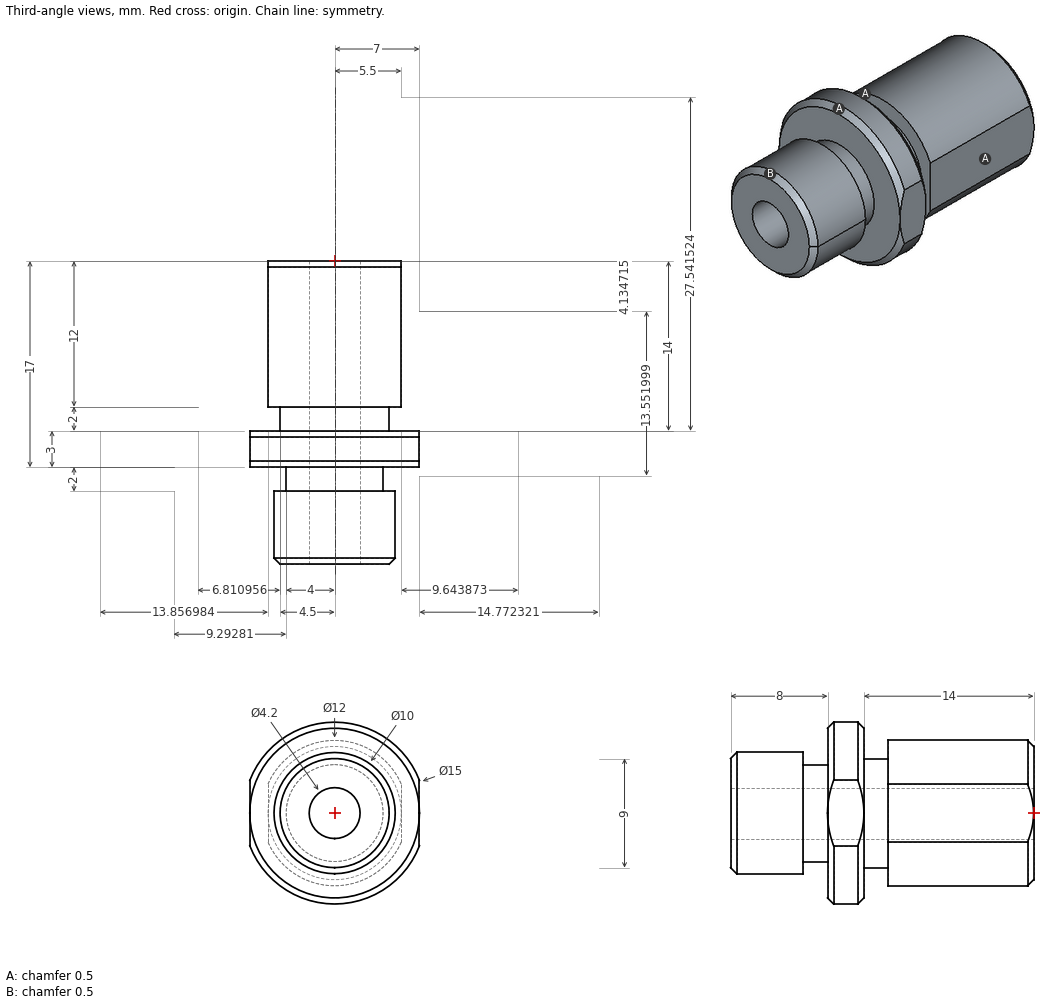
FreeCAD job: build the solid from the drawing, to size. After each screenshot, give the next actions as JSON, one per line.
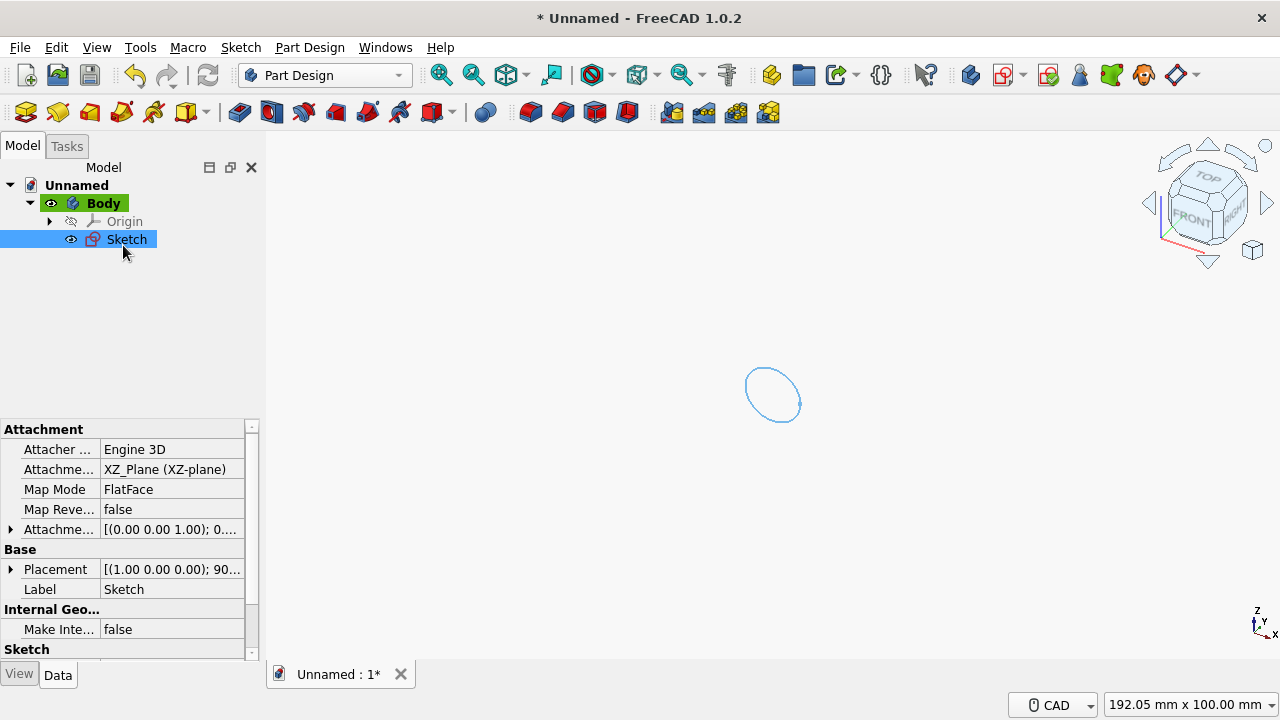
{"action": "left_click", "coordinate": [26, 112]}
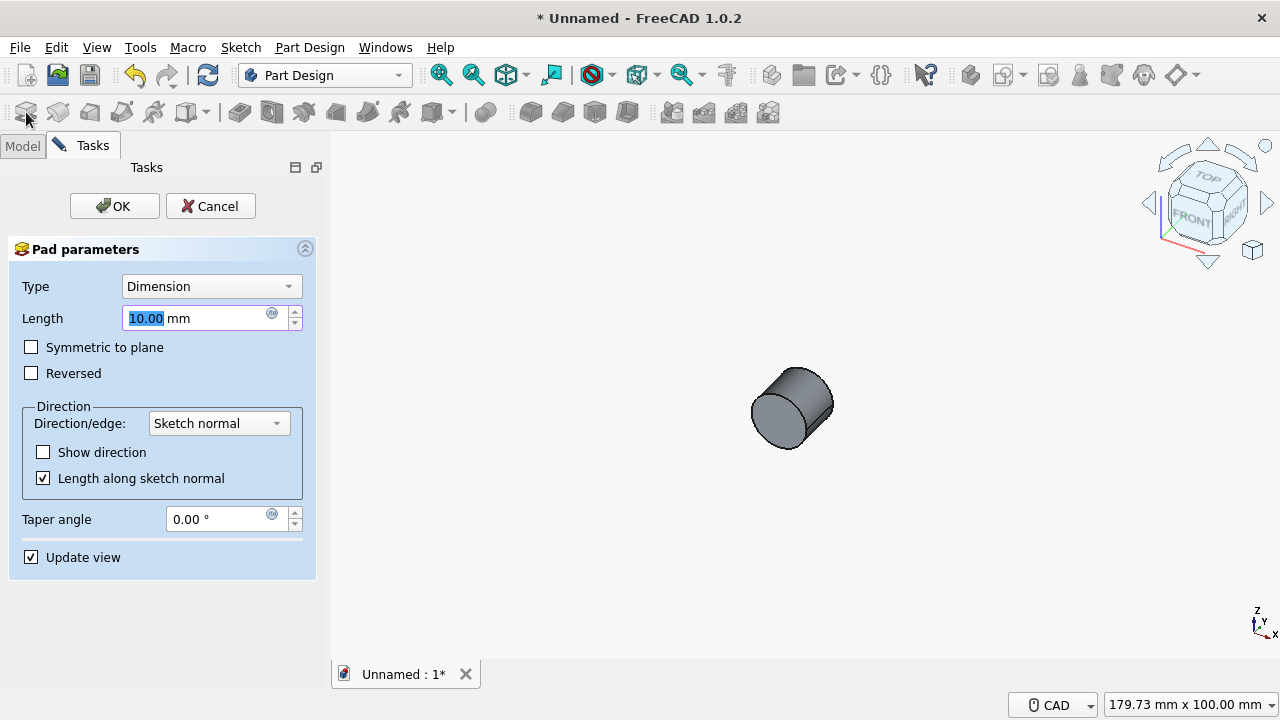
{"action": "type", "text": "14"}
{"action": "key", "text": "Tab"}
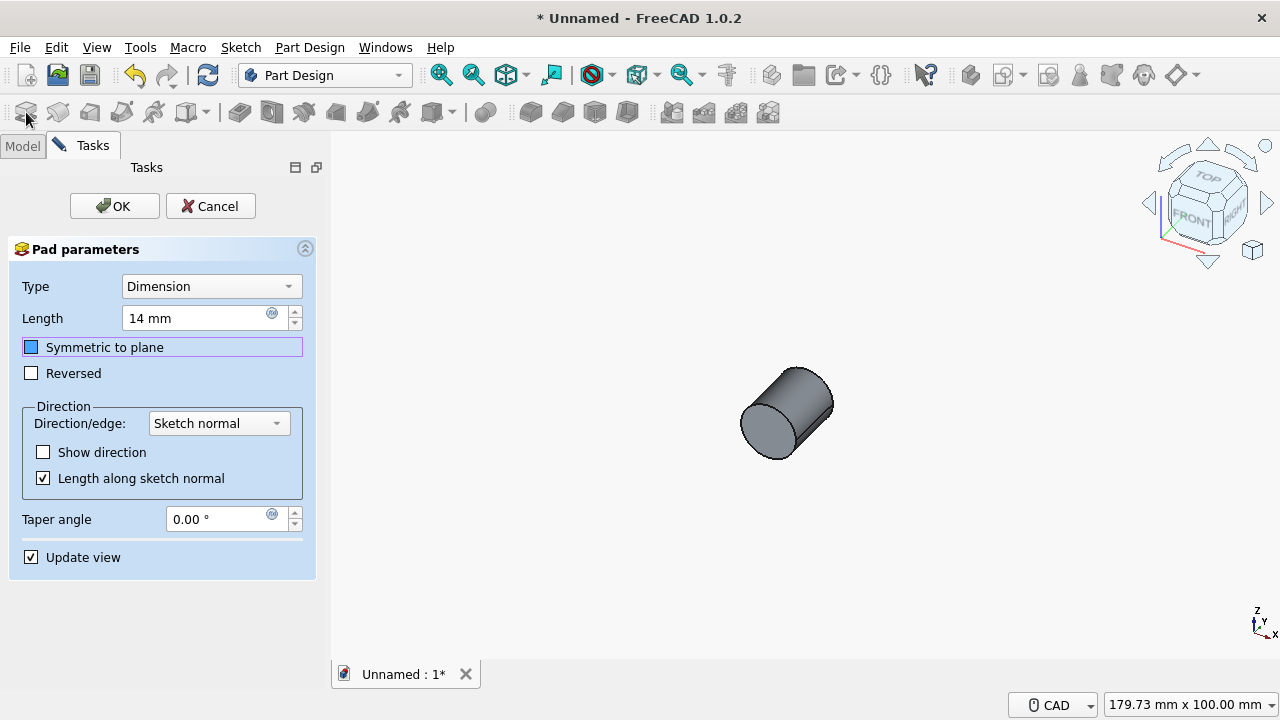
{"action": "left_click", "coordinate": [115, 206]}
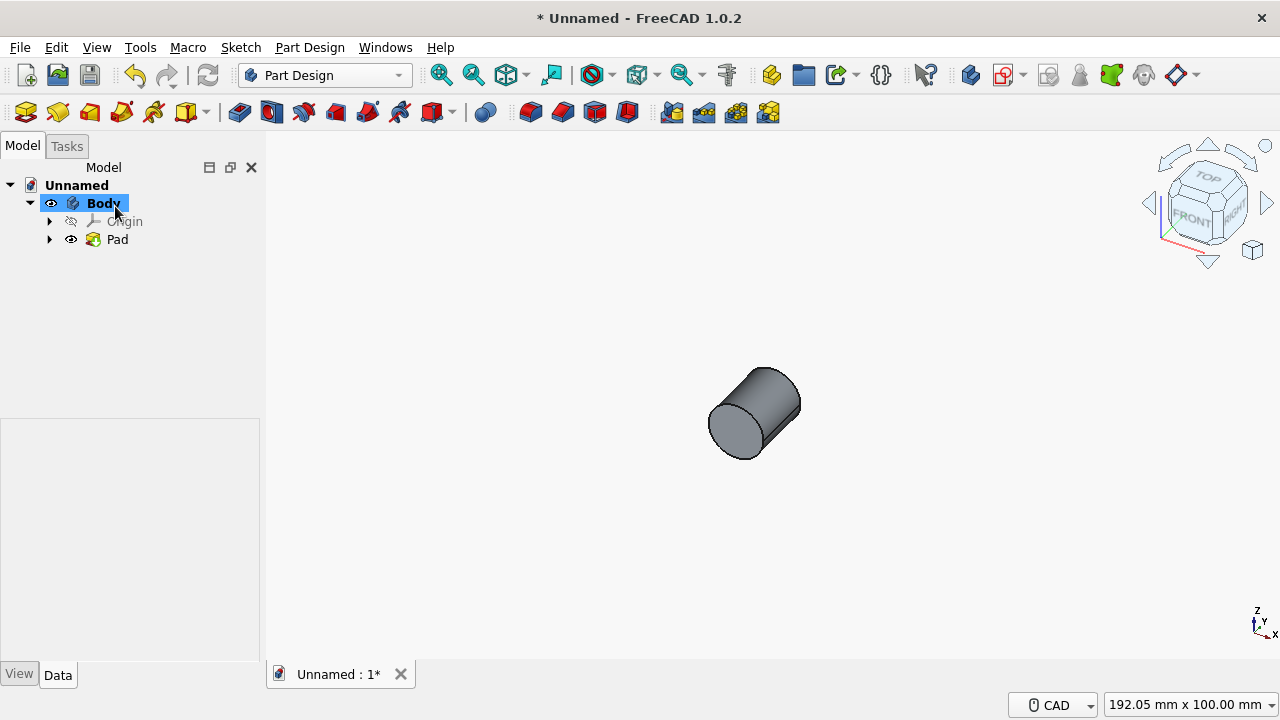
{"action": "key", "text": "v f"}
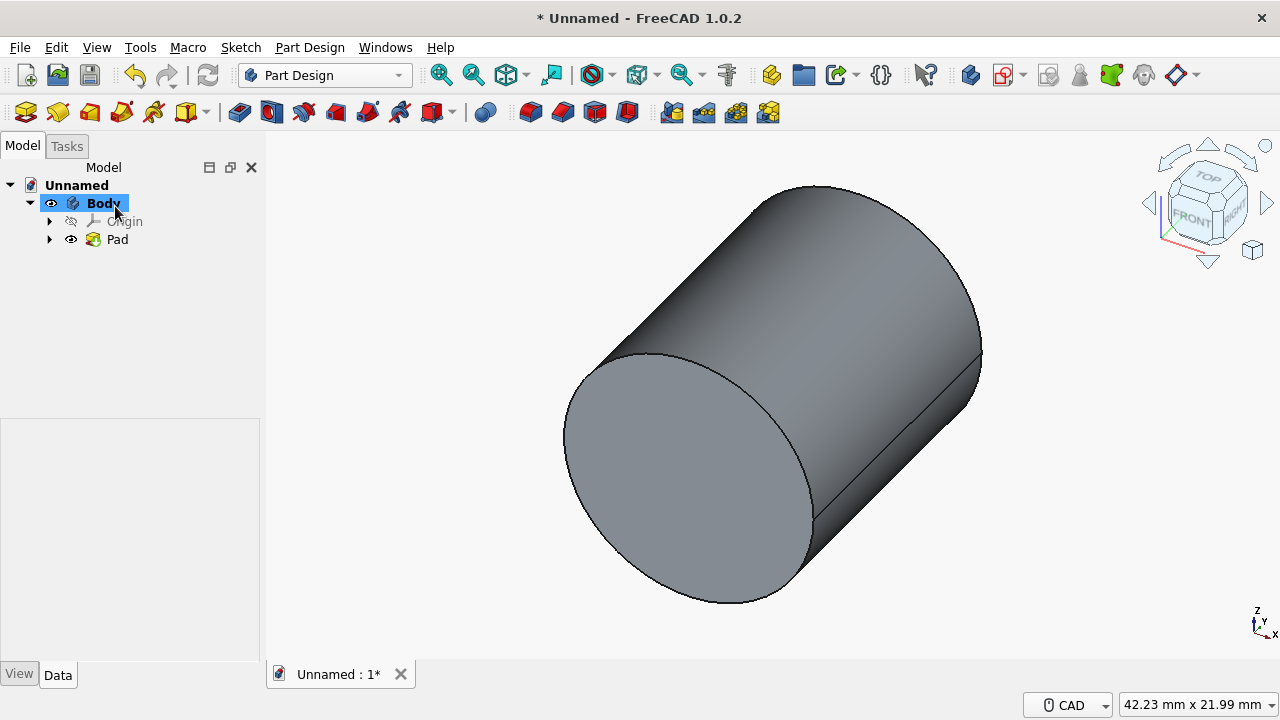
{"action": "left_click", "coordinate": [689, 477]}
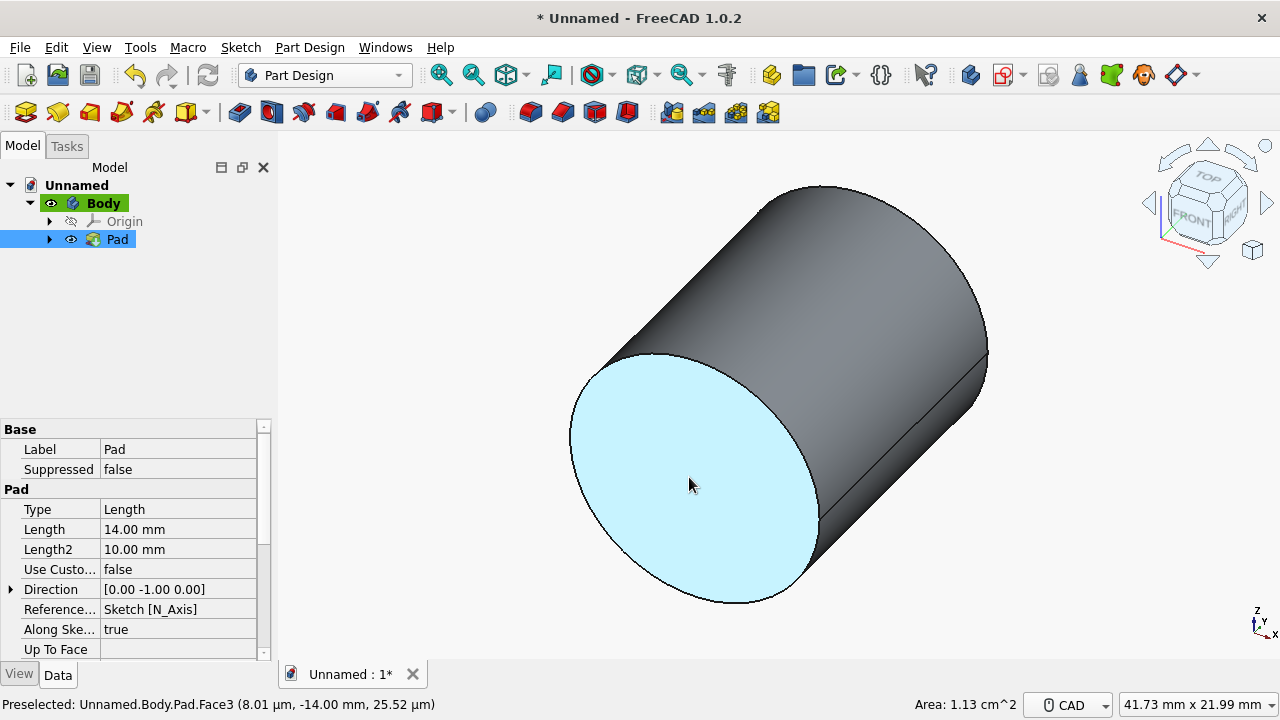
{"action": "left_click", "coordinate": [1004, 76]}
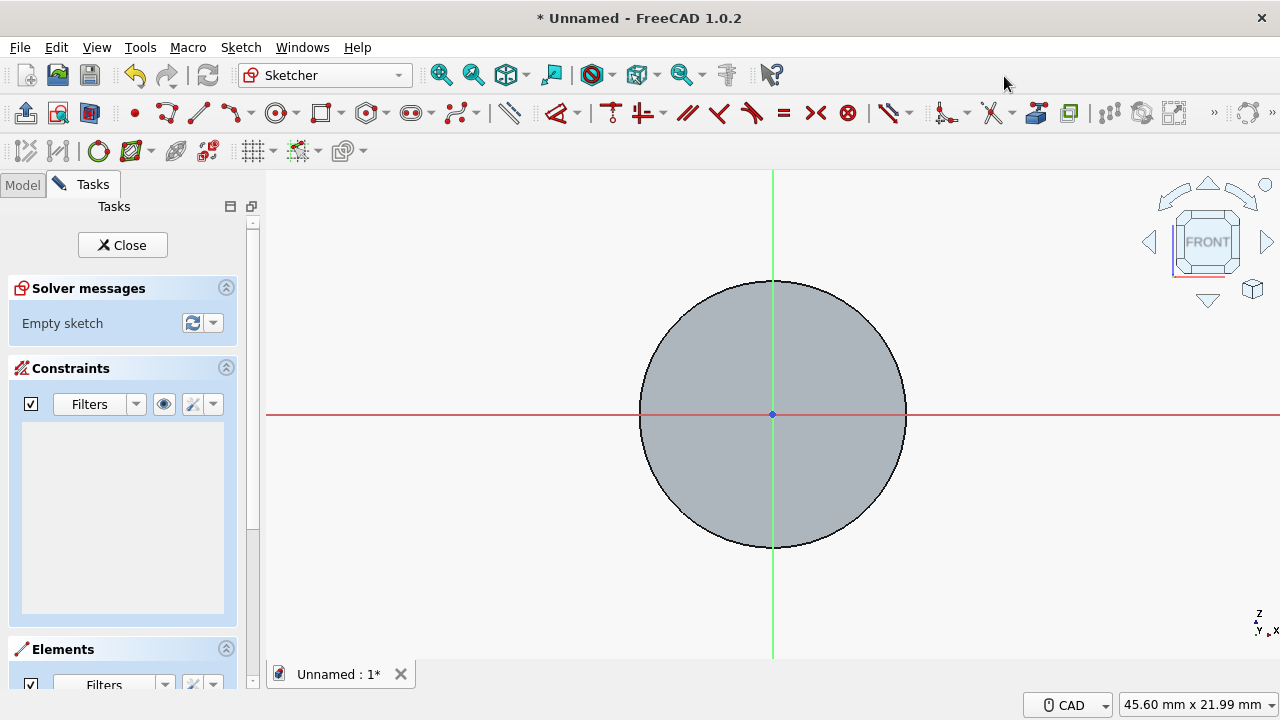
{"action": "key", "text": "g c"}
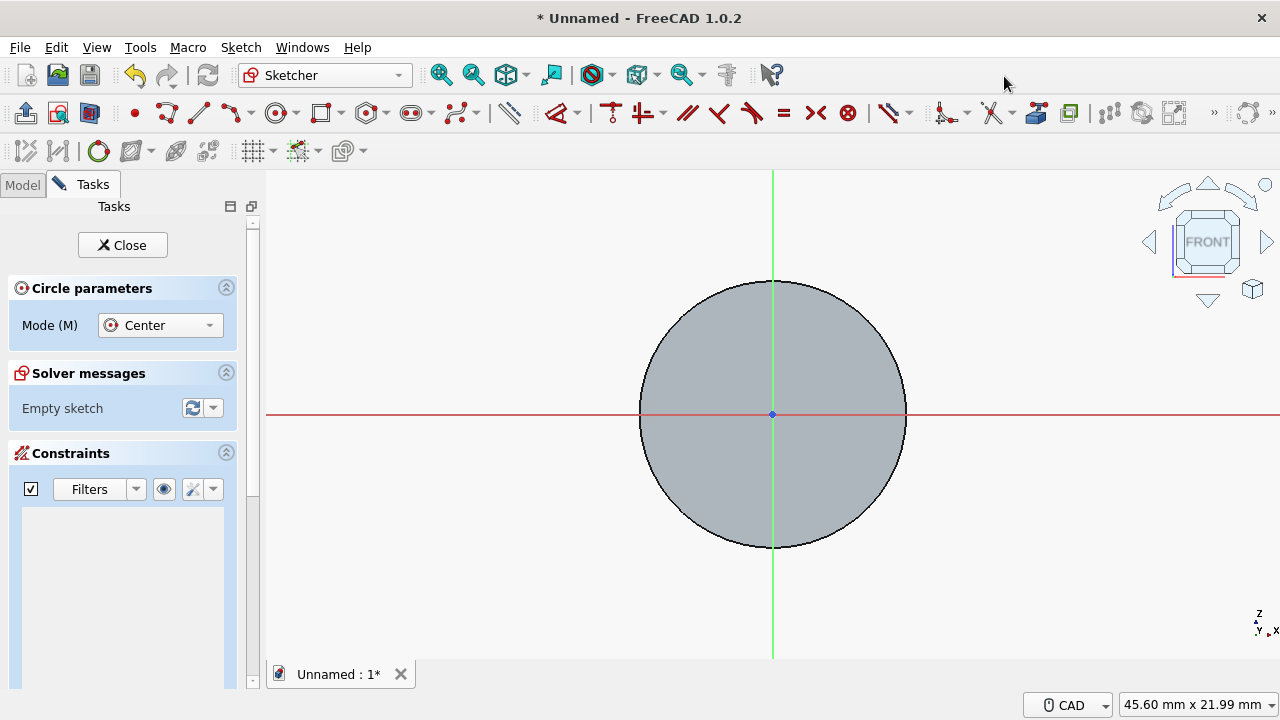
{"action": "left_click", "coordinate": [773, 414]}
{"action": "left_click", "coordinate": [891, 297]}
{"action": "key", "text": "Escape"}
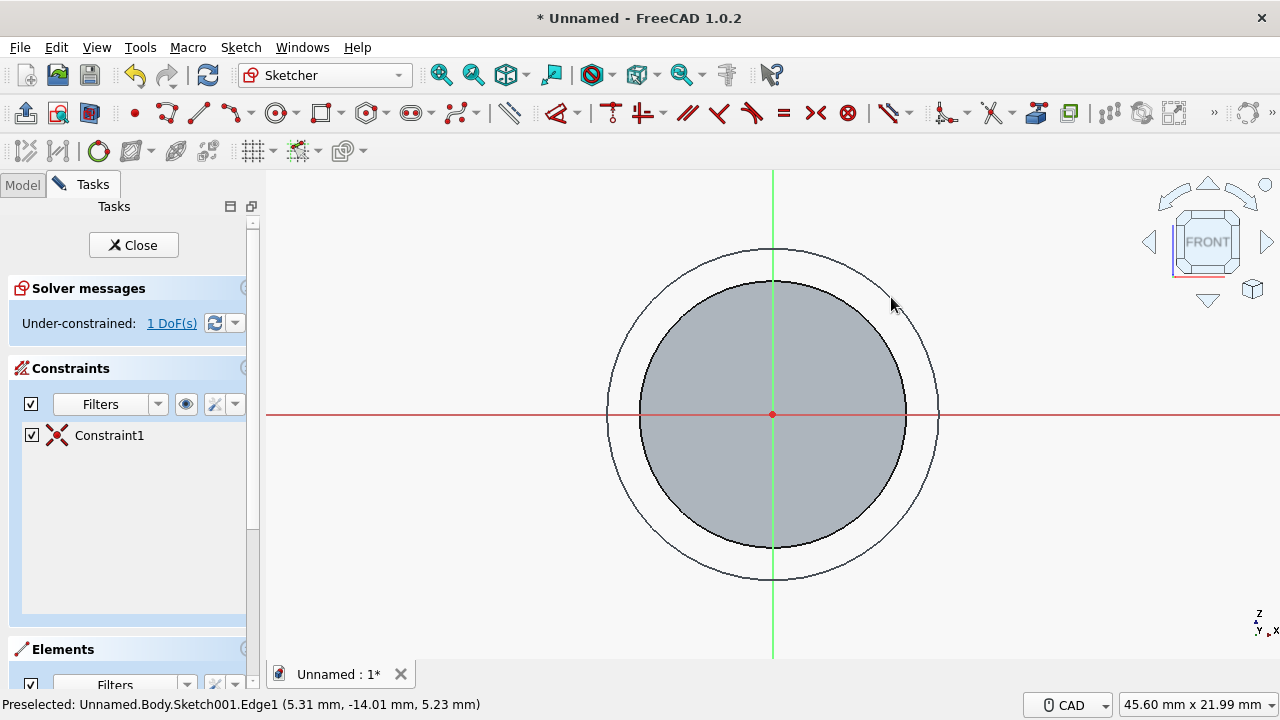
{"action": "left_click", "coordinate": [556, 114]}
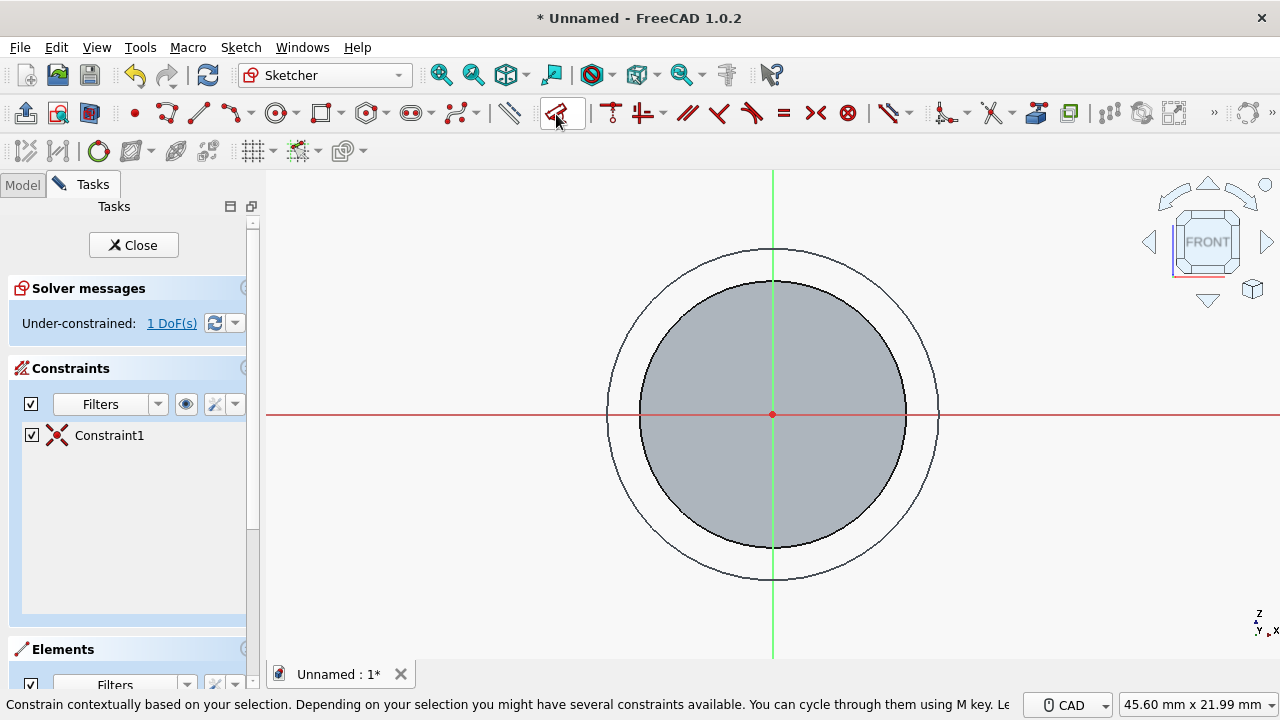
{"action": "left_click", "coordinate": [890, 297]}
{"action": "left_click", "coordinate": [913, 274]}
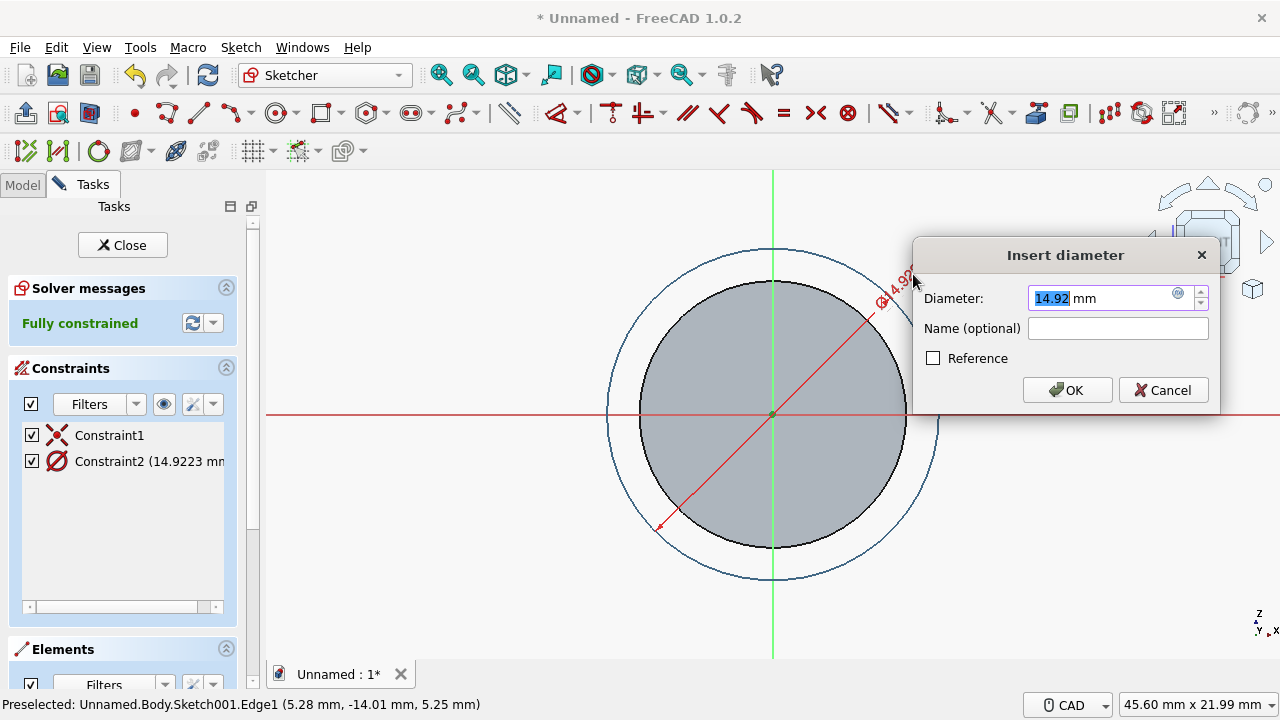
{"action": "type", "text": "15"}
{"action": "key", "text": "Return"}
{"action": "key", "text": "Escape"}